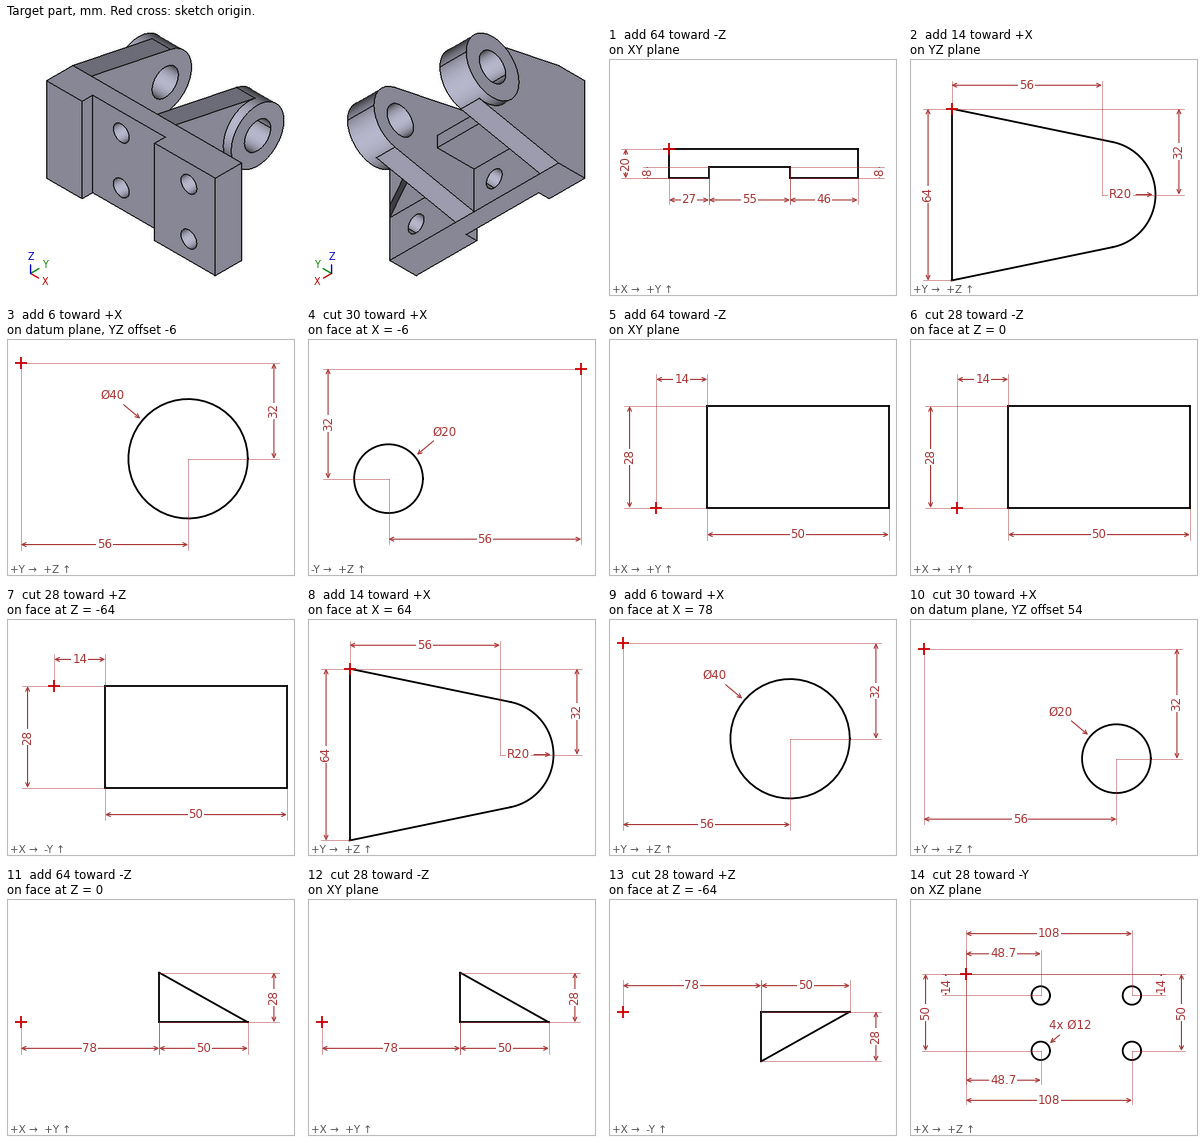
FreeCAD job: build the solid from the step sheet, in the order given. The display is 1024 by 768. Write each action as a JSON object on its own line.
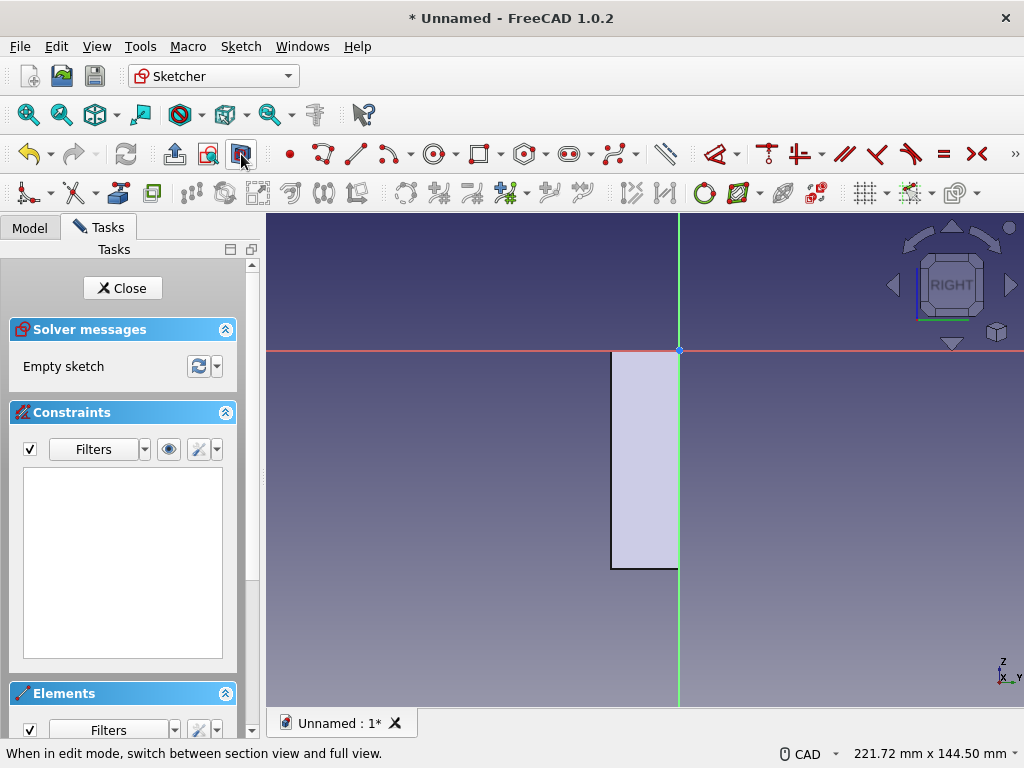
{"action": "scroll", "coordinate": [294, 460], "scroll_direction": "down", "scroll_amount": 1}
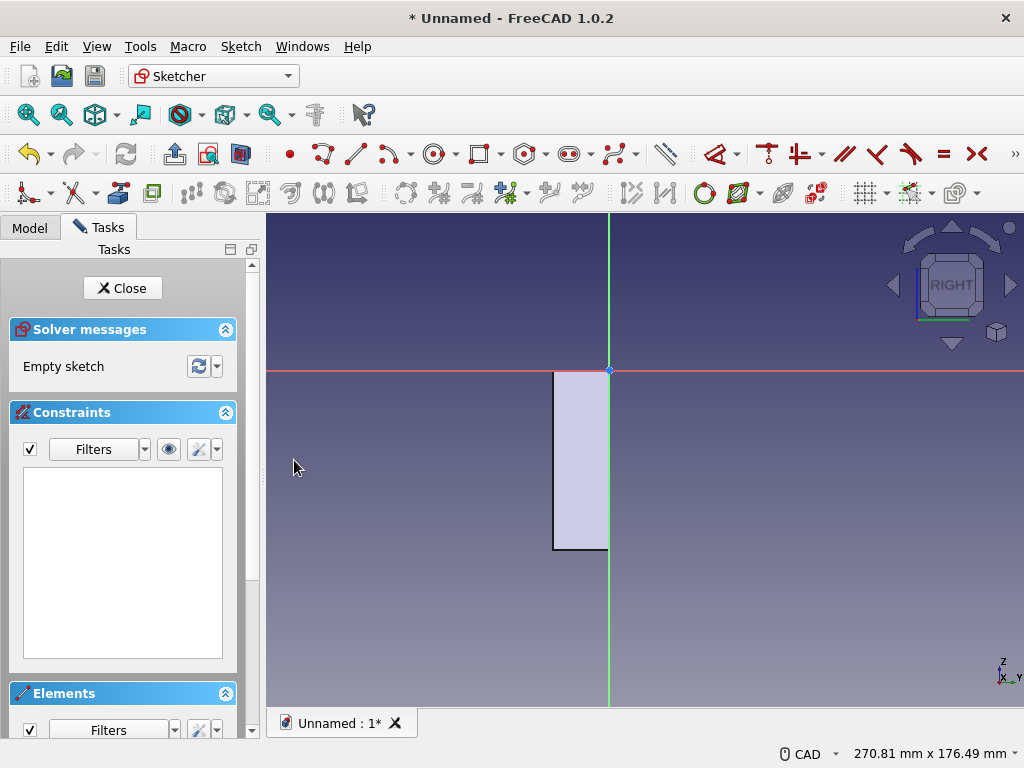
{"action": "scroll", "coordinate": [859, 460], "scroll_direction": "up", "scroll_amount": 3}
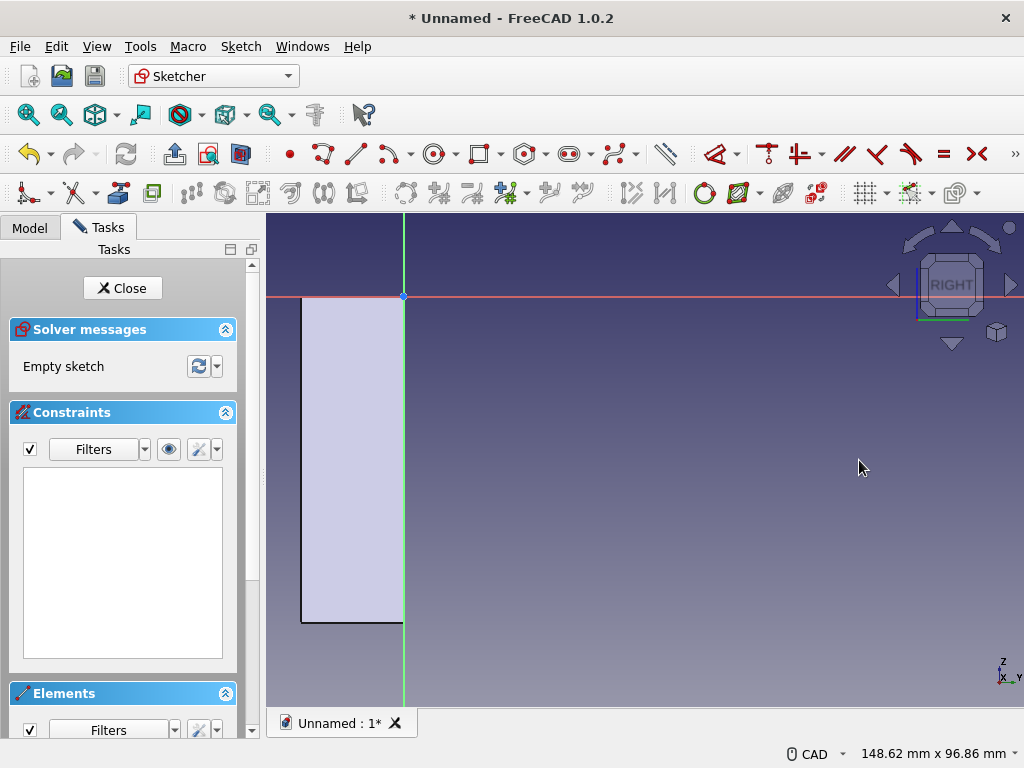
{"action": "left_click", "coordinate": [323, 154]}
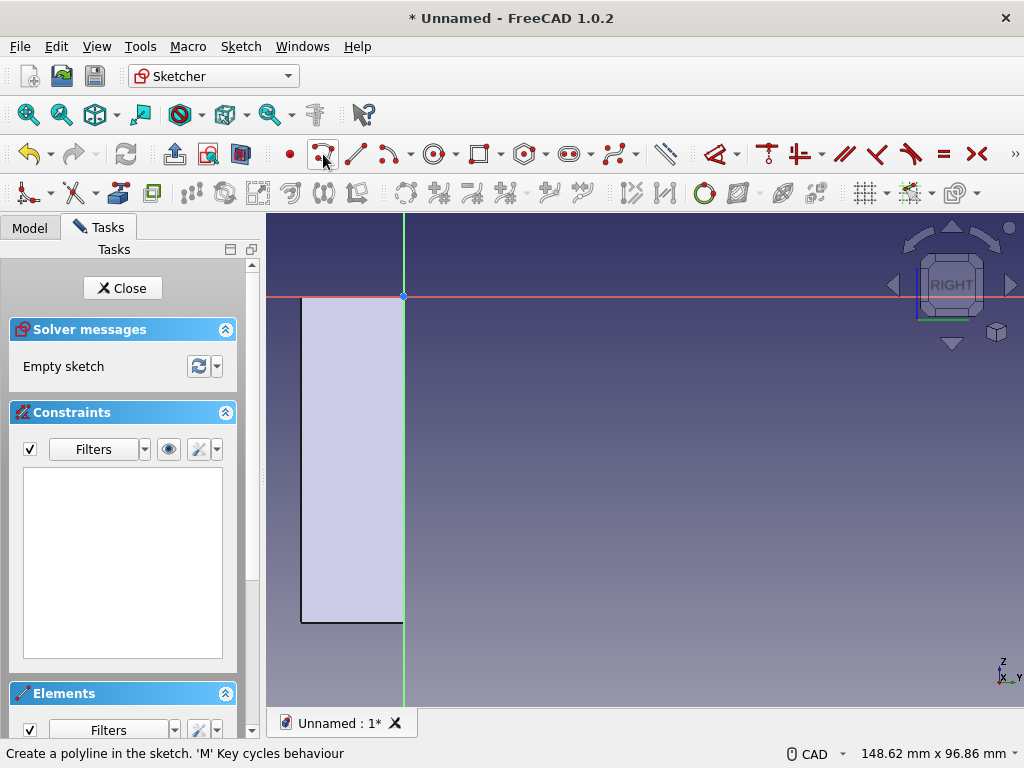
{"action": "left_click", "coordinate": [710, 560]}
{"action": "left_click", "coordinate": [404, 623]}
{"action": "left_click", "coordinate": [404, 297]}
{"action": "left_click", "coordinate": [710, 360]}
{"action": "right_click", "coordinate": [710, 360]}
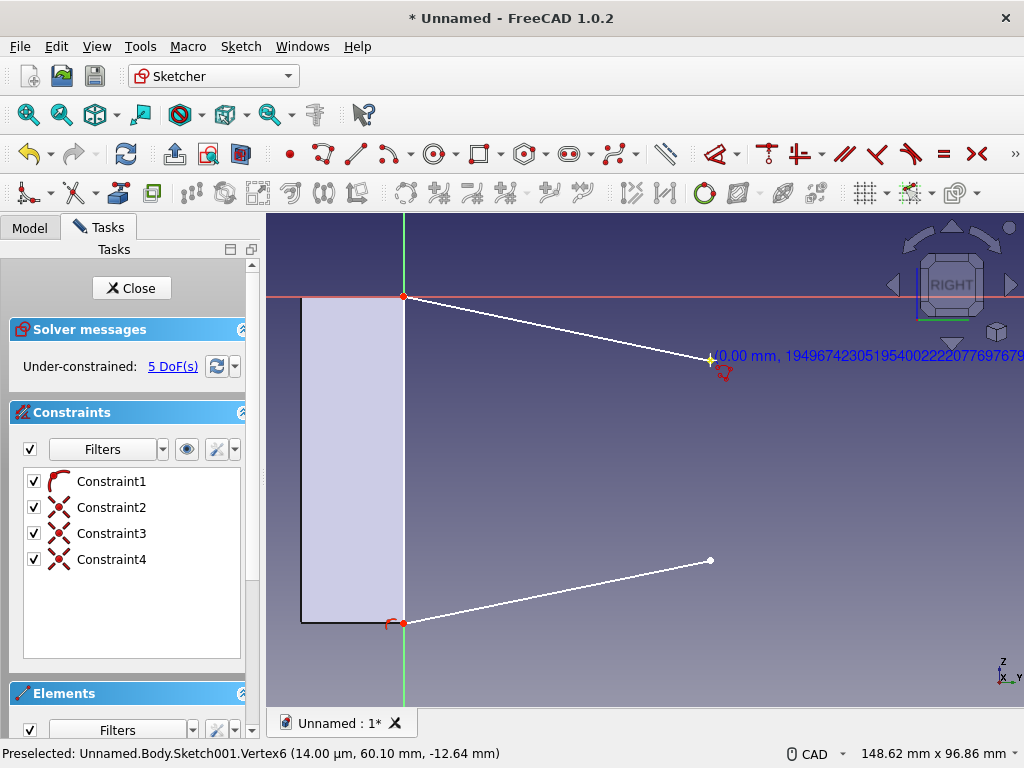
{"action": "left_click", "coordinate": [410, 154]}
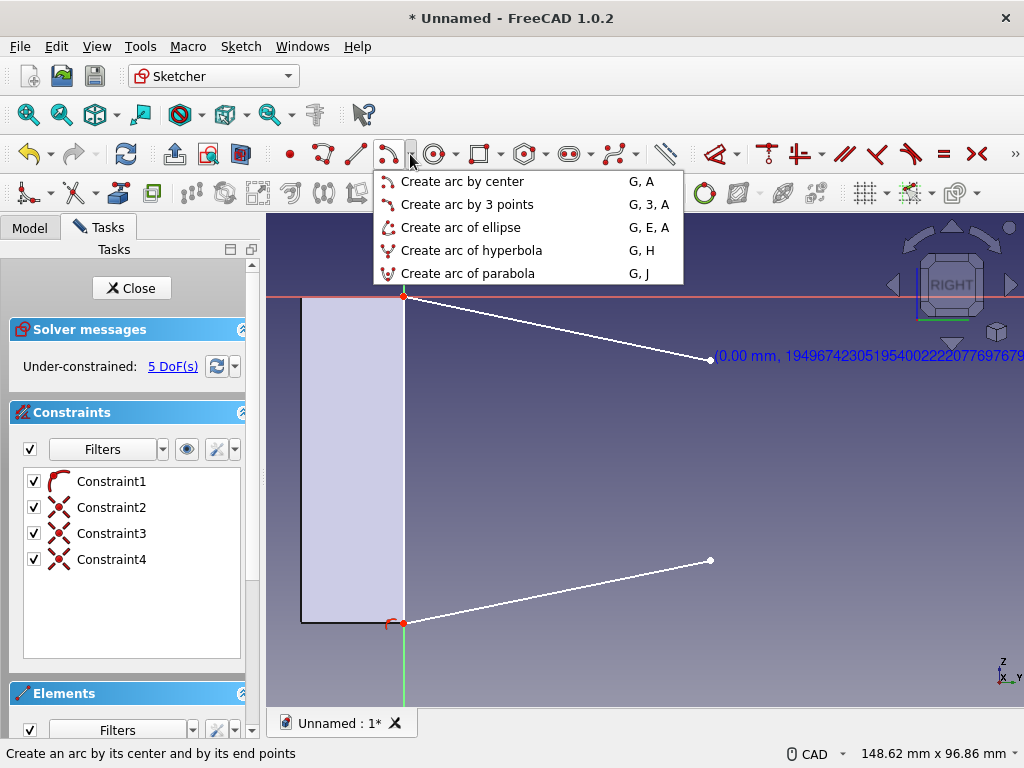
{"action": "left_click", "coordinate": [528, 204]}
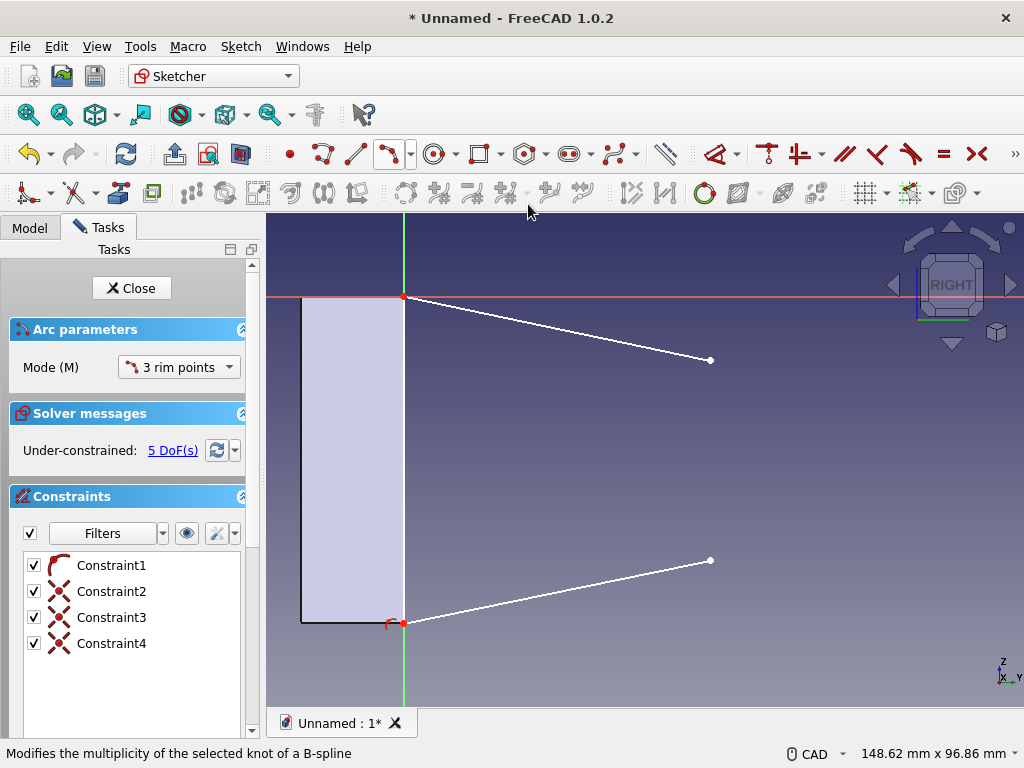
{"action": "left_click", "coordinate": [710, 361]}
{"action": "left_click", "coordinate": [710, 561]}
{"action": "left_click", "coordinate": [791, 460]}
{"action": "key", "text": "Escape"}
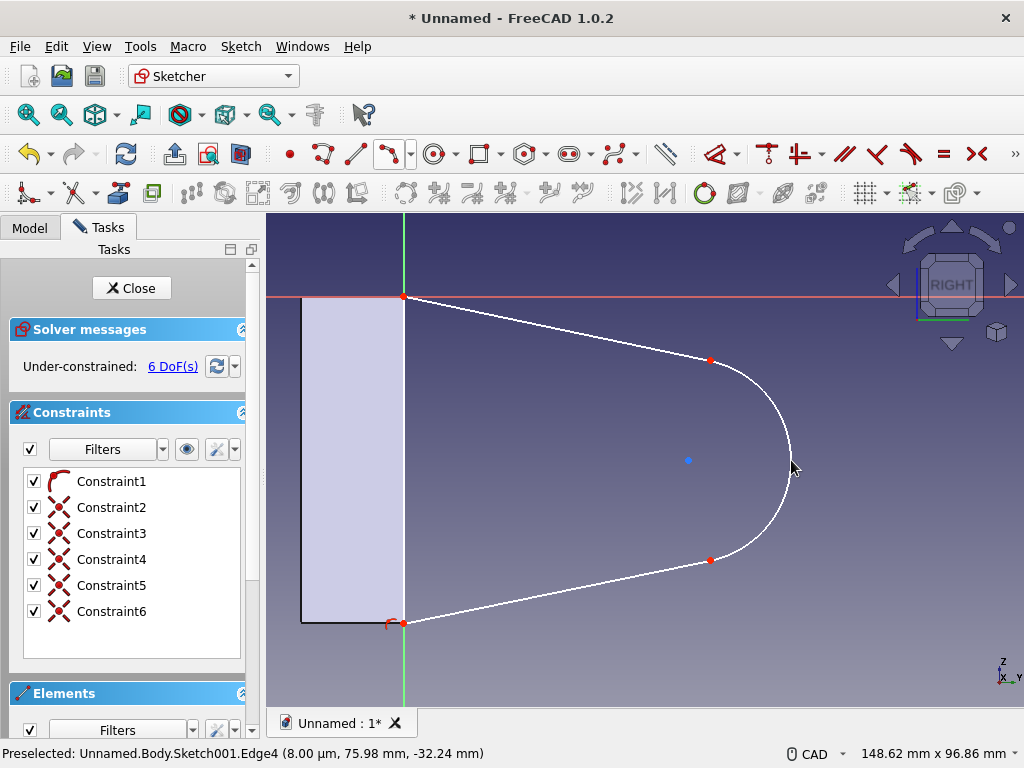
{"action": "left_click", "coordinate": [618, 580]}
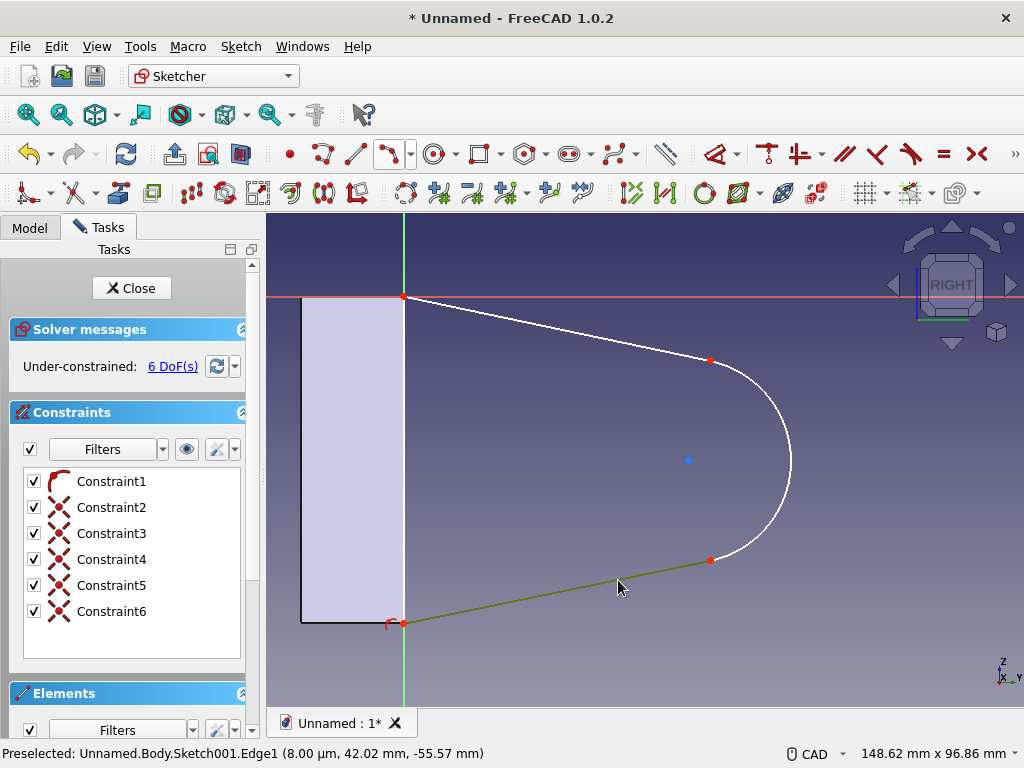
{"action": "left_click", "coordinate": [776, 514]}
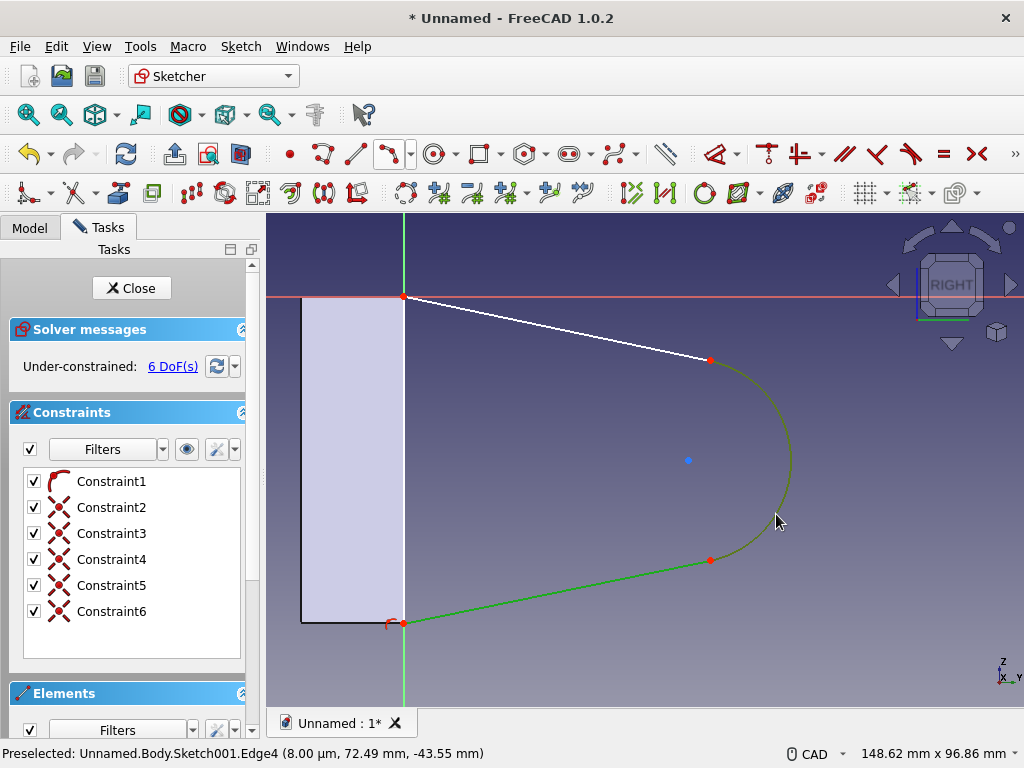
{"action": "left_click", "coordinate": [911, 154]}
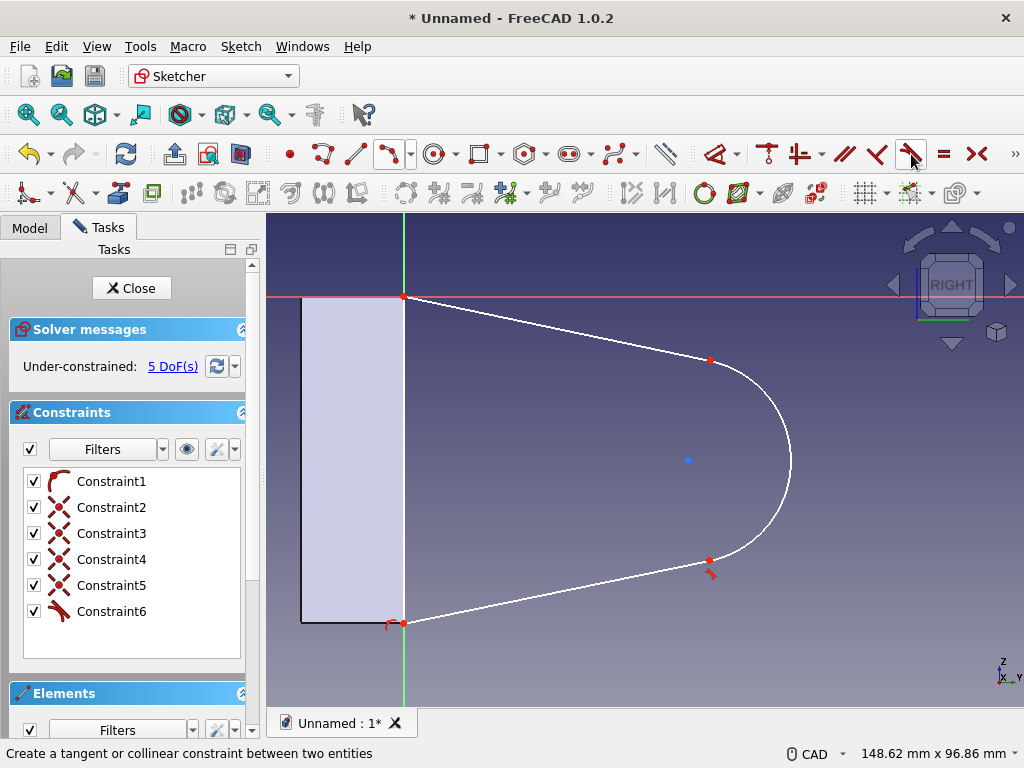
{"action": "left_click", "coordinate": [495, 316]}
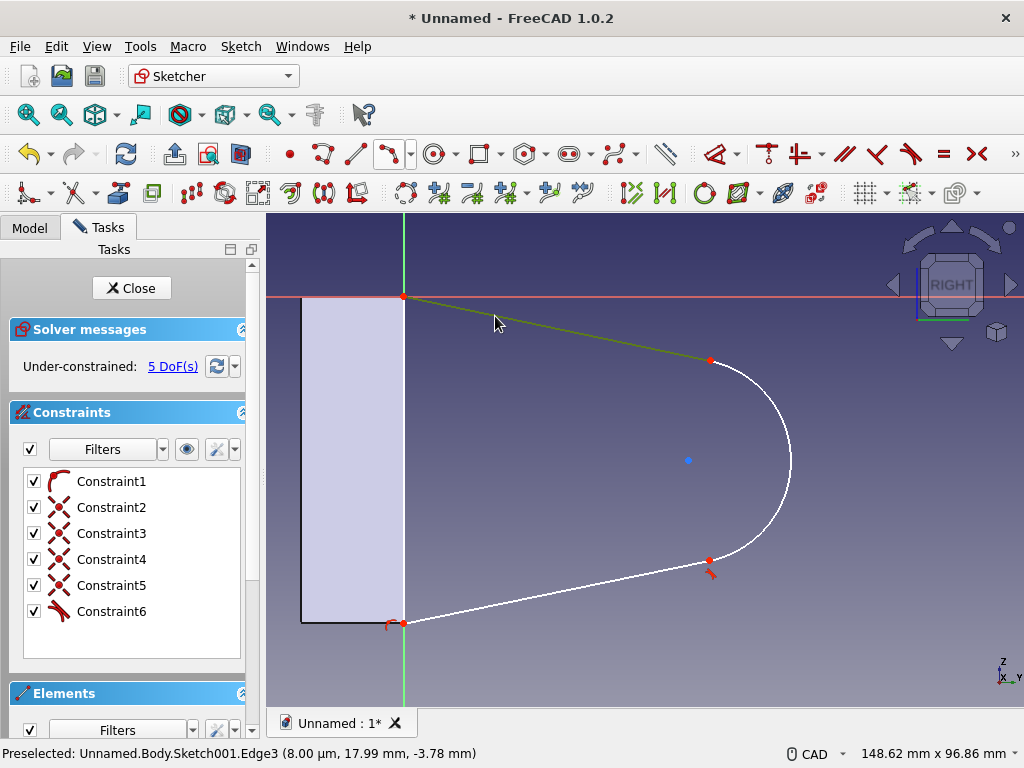
{"action": "left_click", "coordinate": [776, 514]}